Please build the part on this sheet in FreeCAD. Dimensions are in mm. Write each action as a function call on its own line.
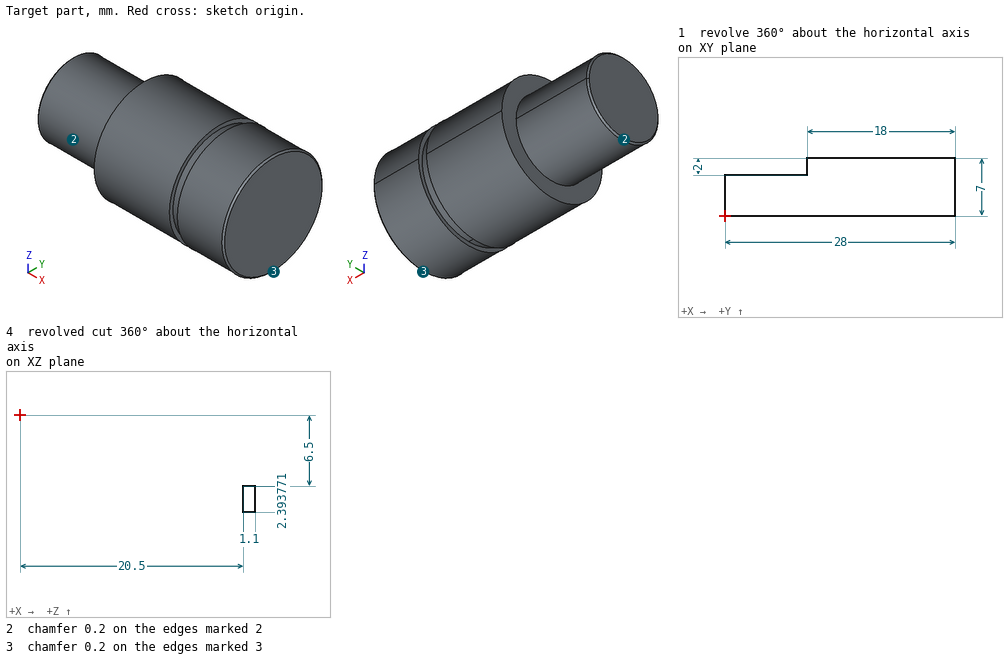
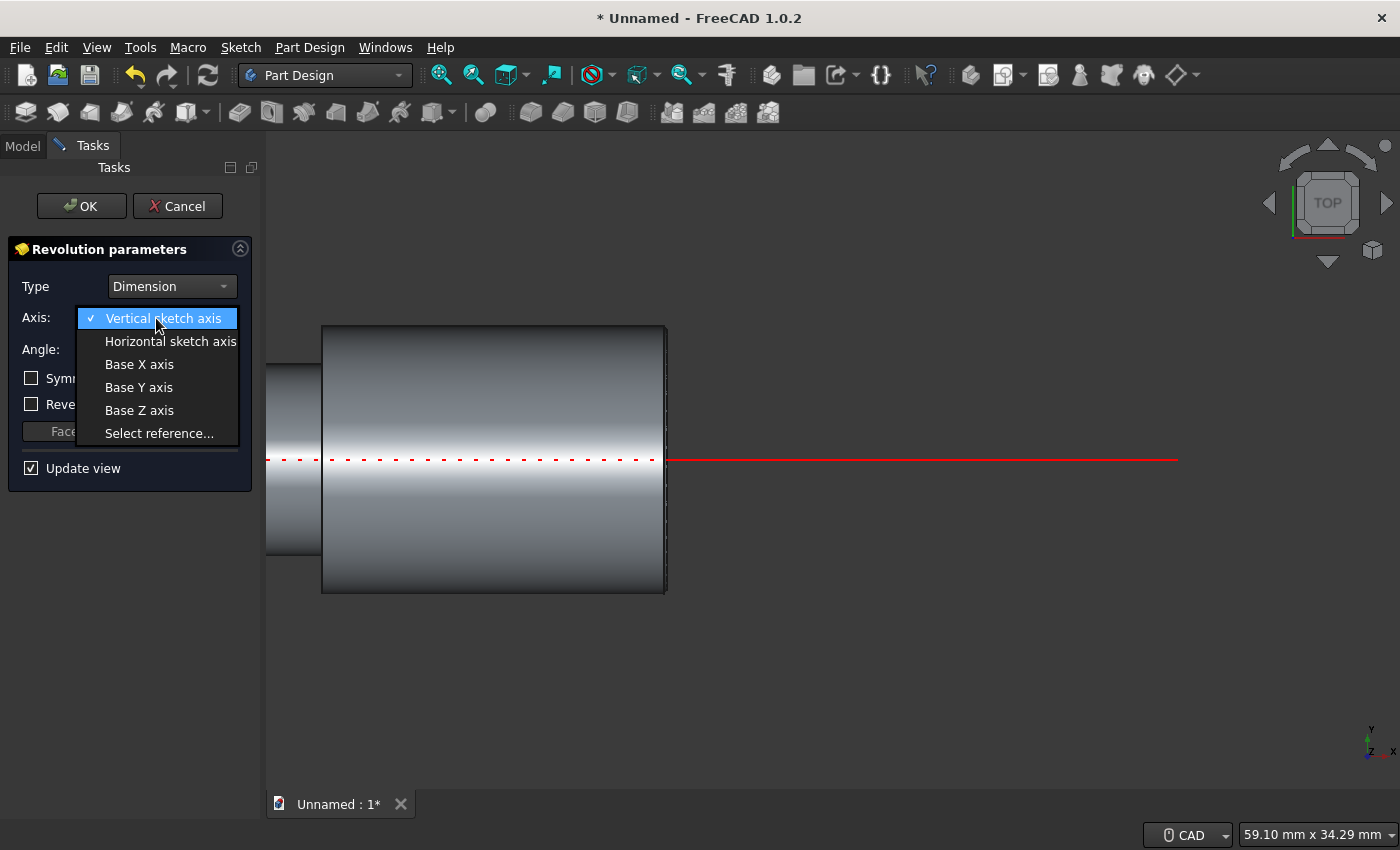
click(156, 342)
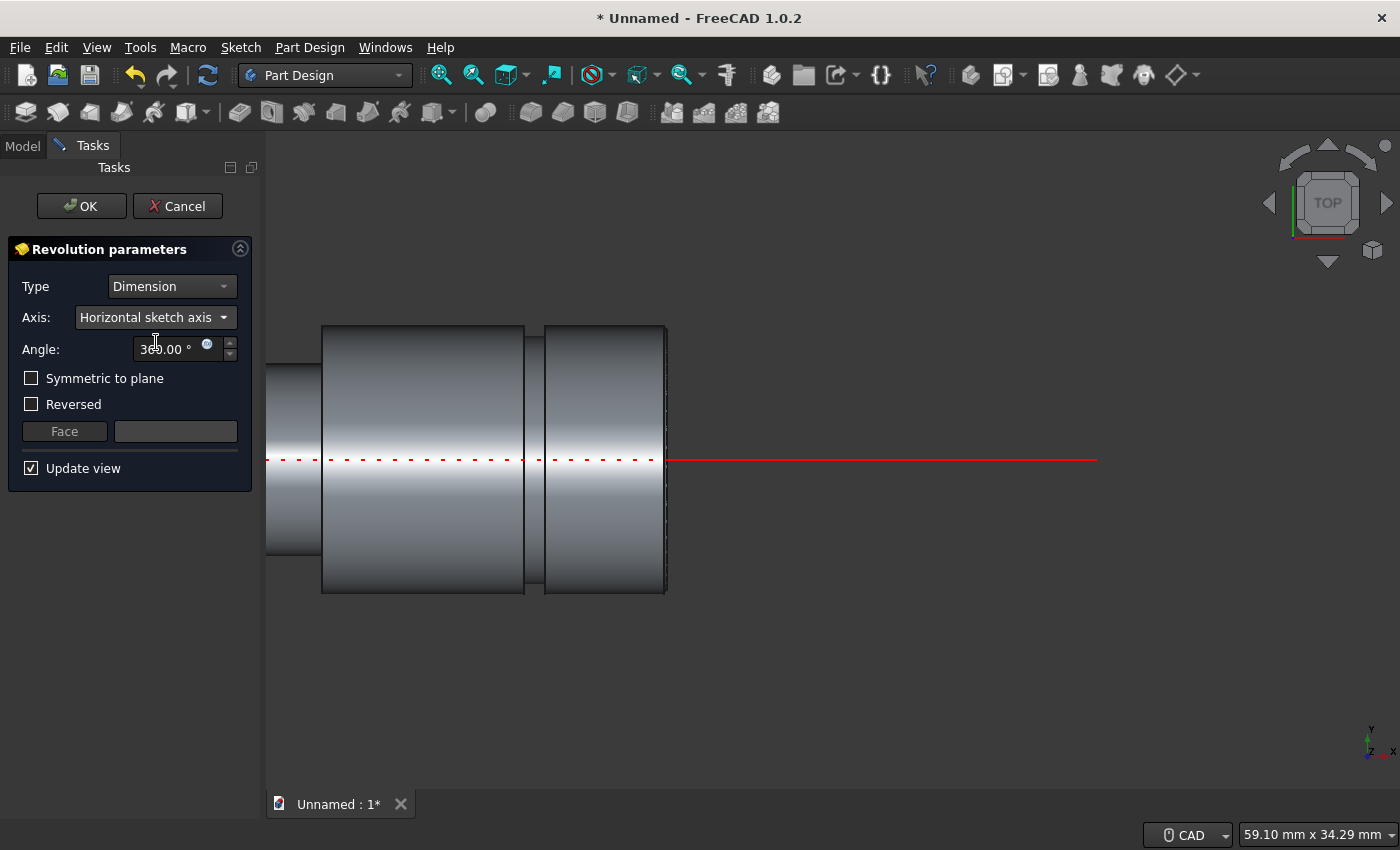
click(82, 206)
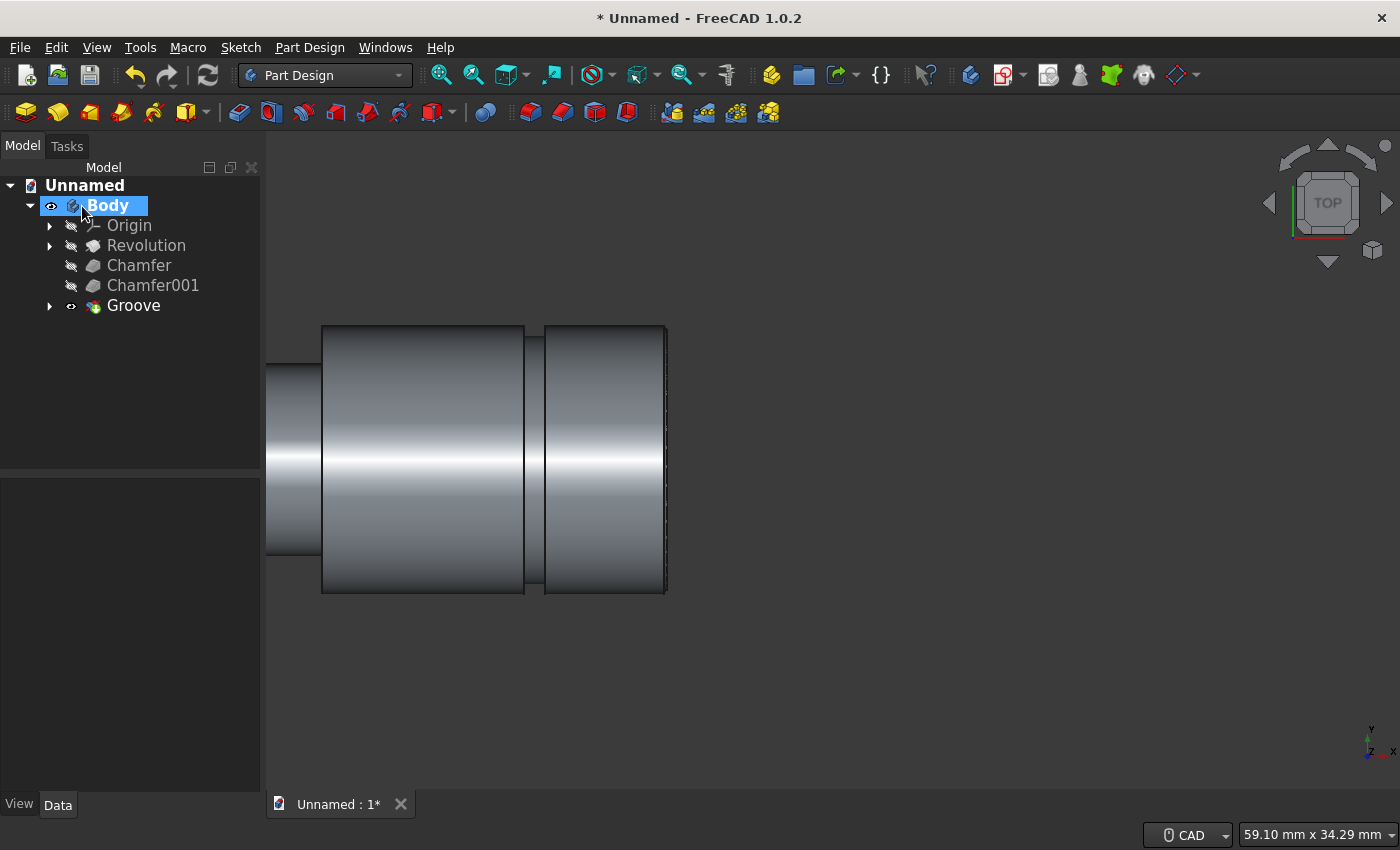
key(0)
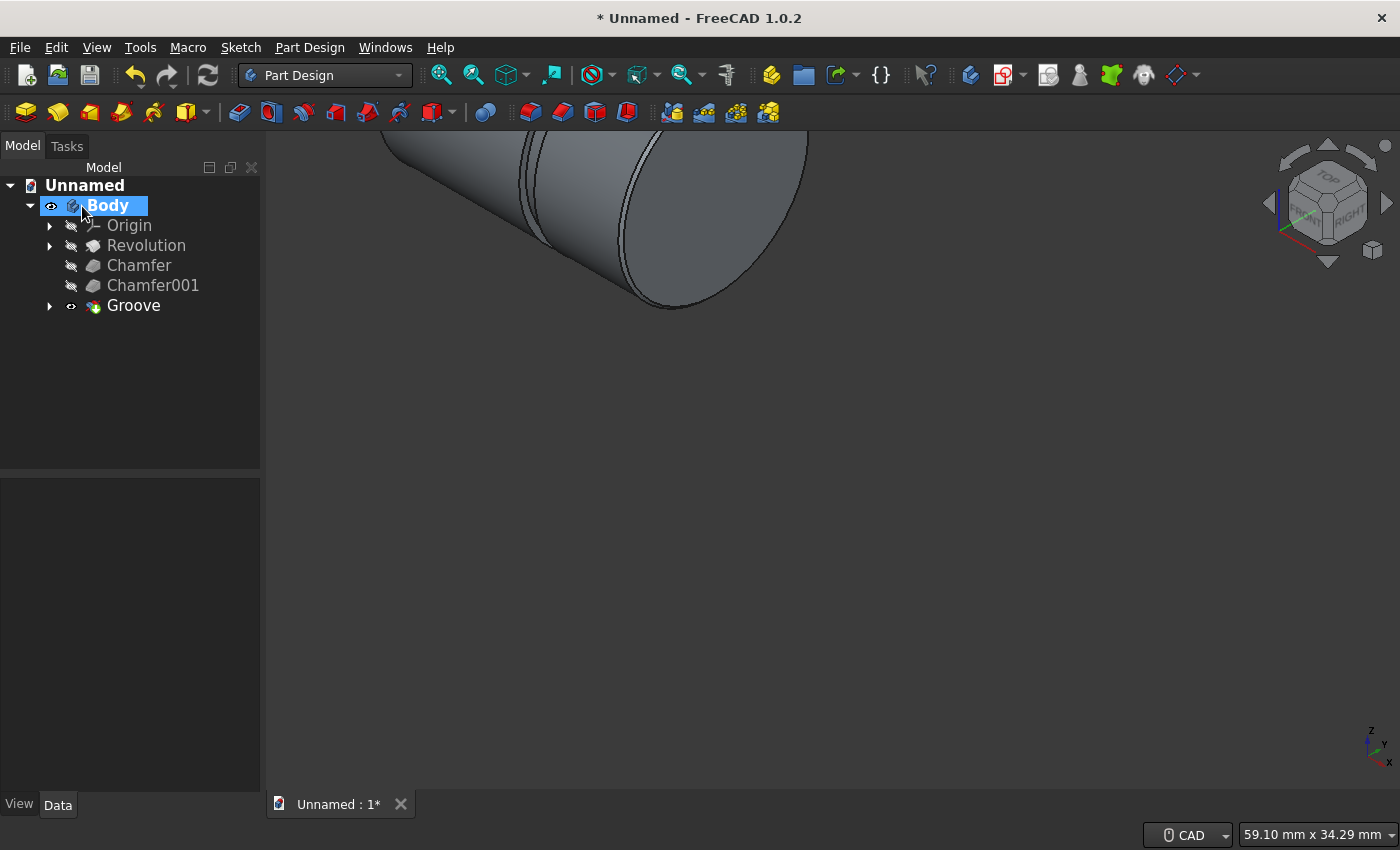
click(442, 76)